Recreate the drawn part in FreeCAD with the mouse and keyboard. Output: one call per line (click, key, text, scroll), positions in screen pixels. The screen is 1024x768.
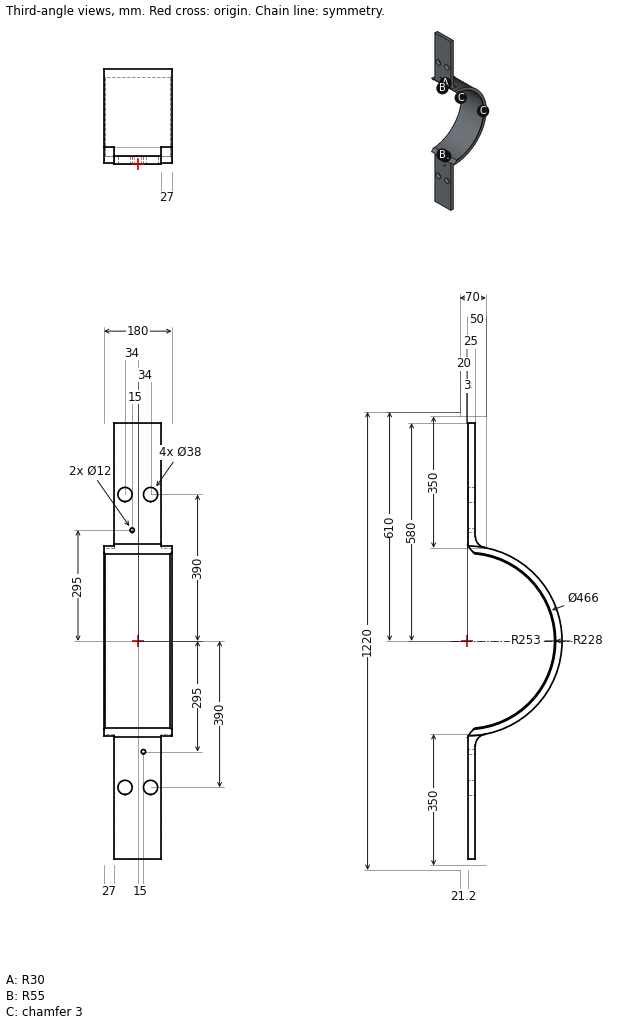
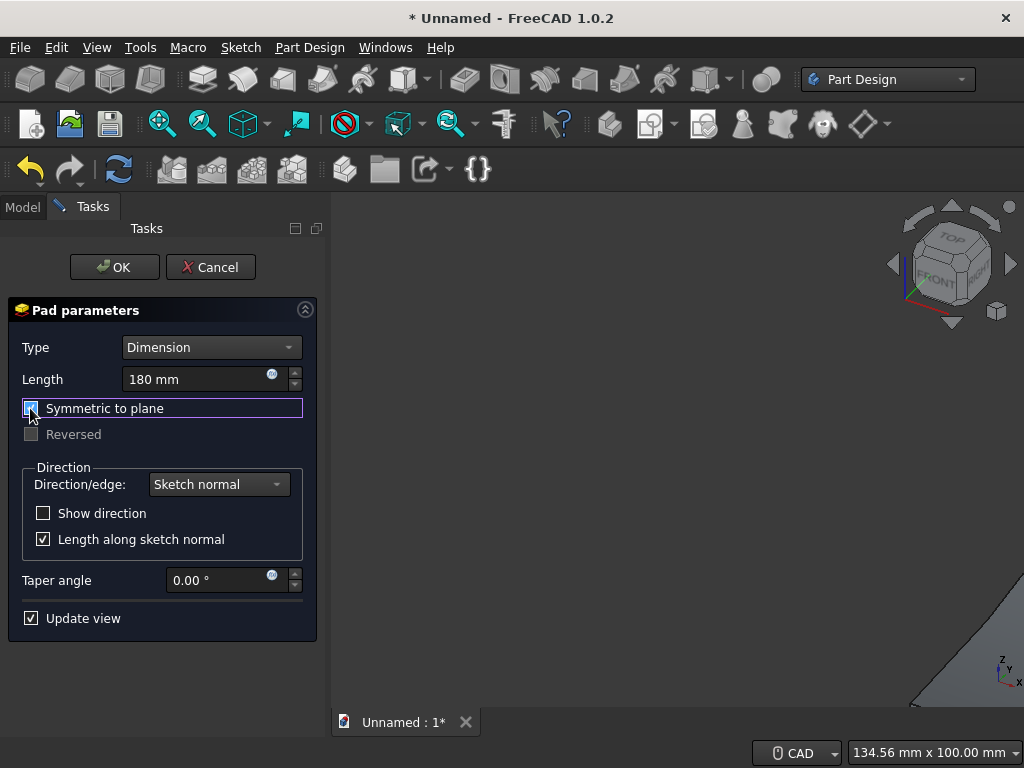
click(115, 267)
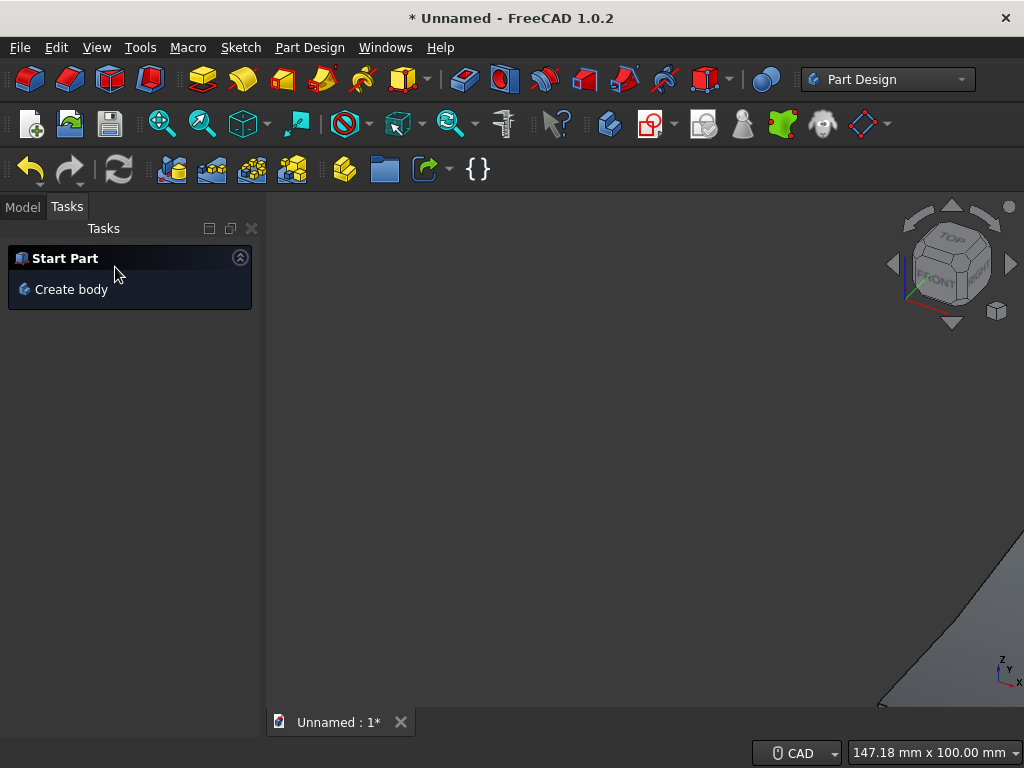
click(164, 124)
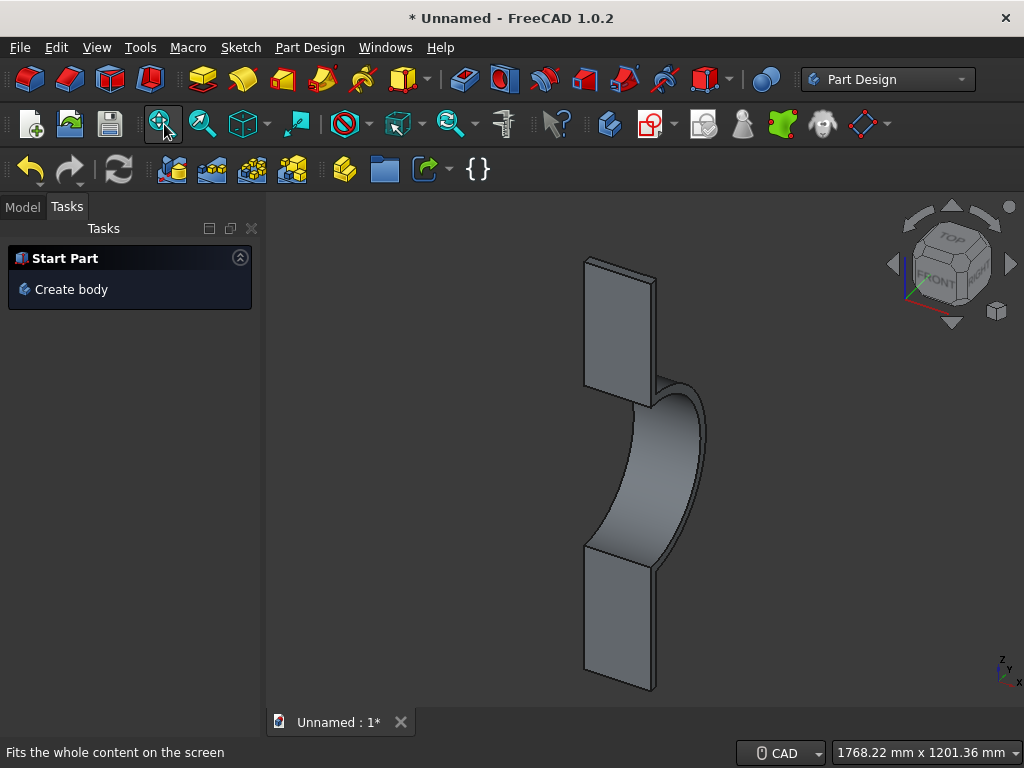
key(0)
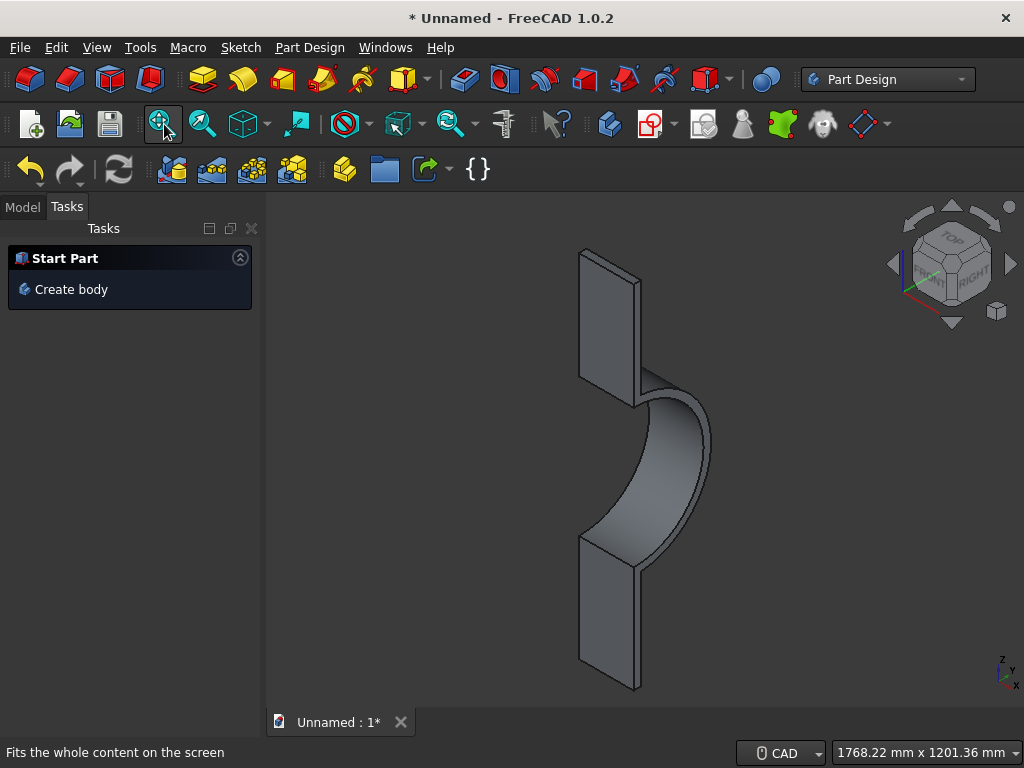
key(2)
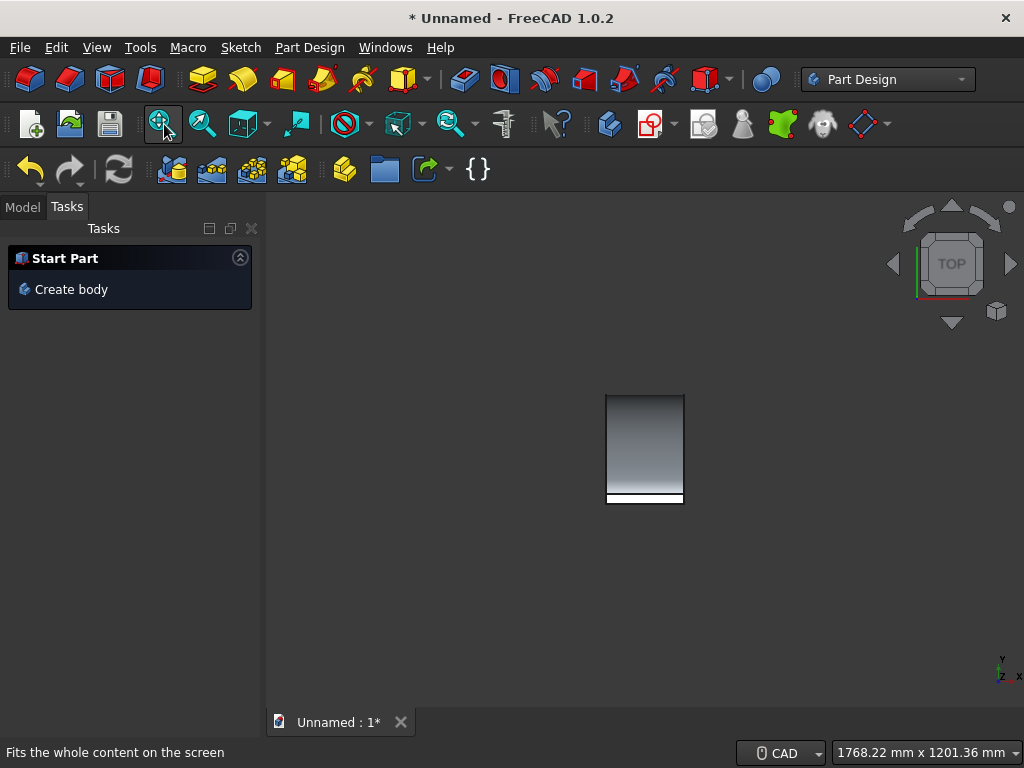
click(164, 124)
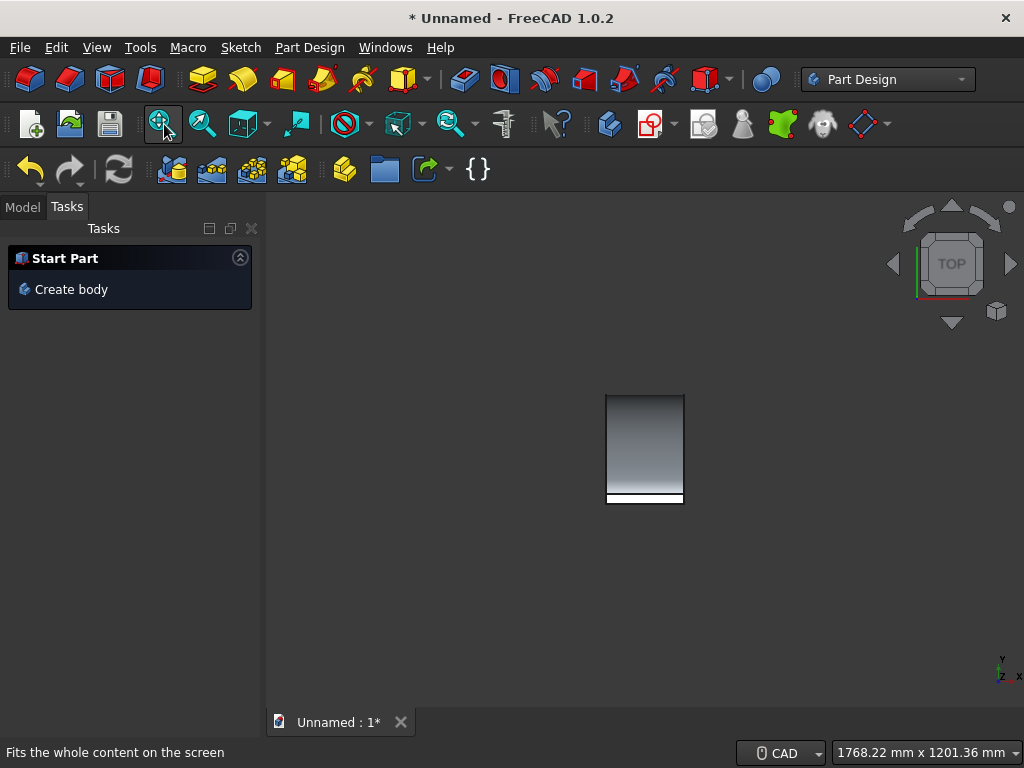
key(1)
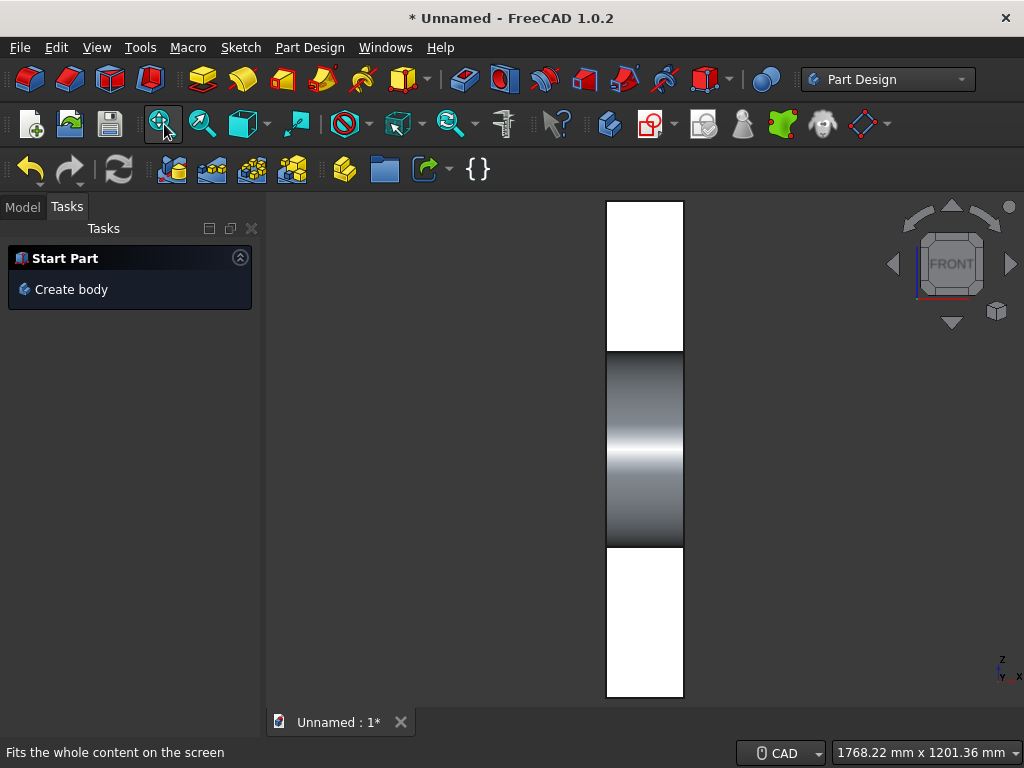
key(3)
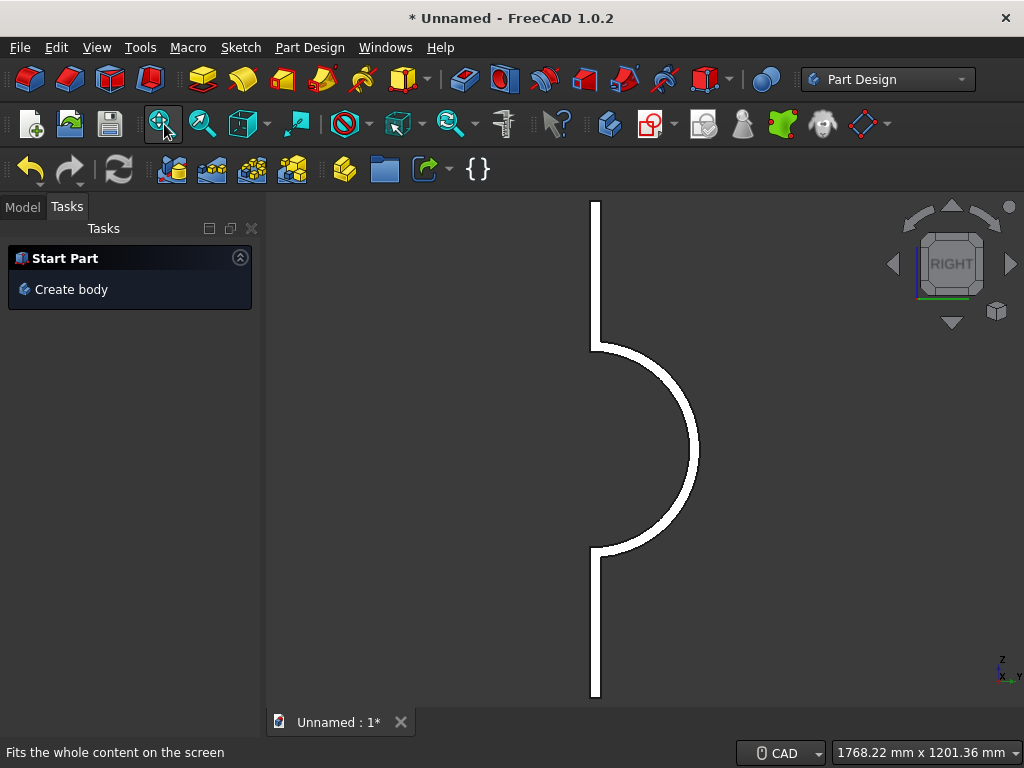
key(5)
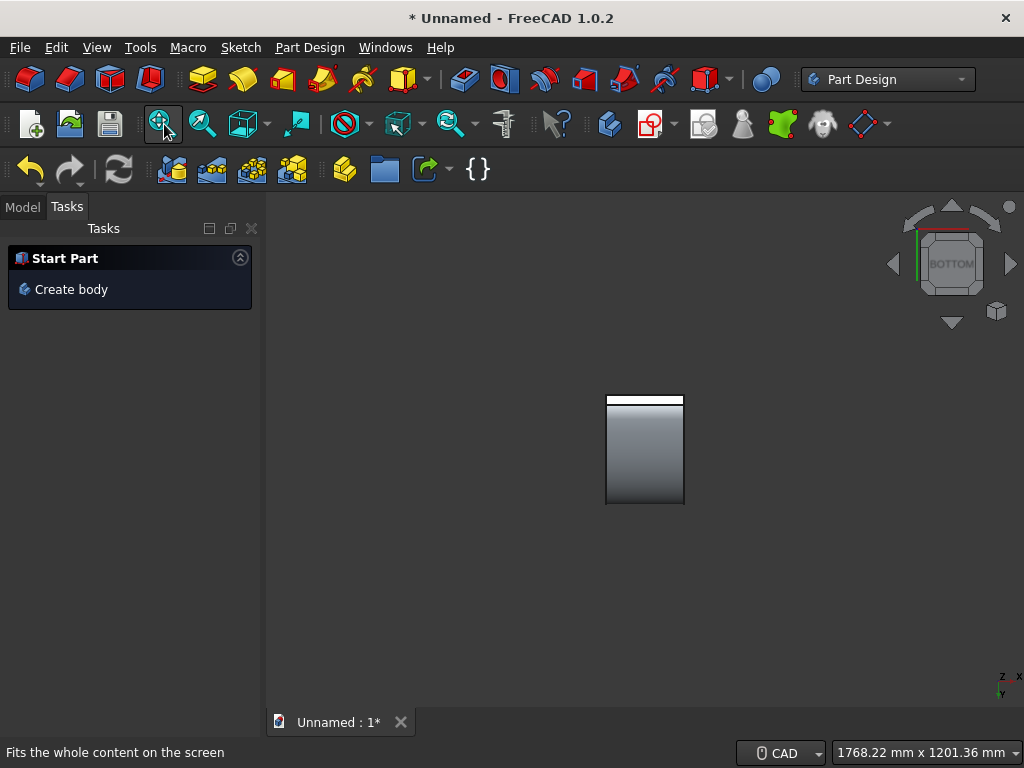
click(164, 124)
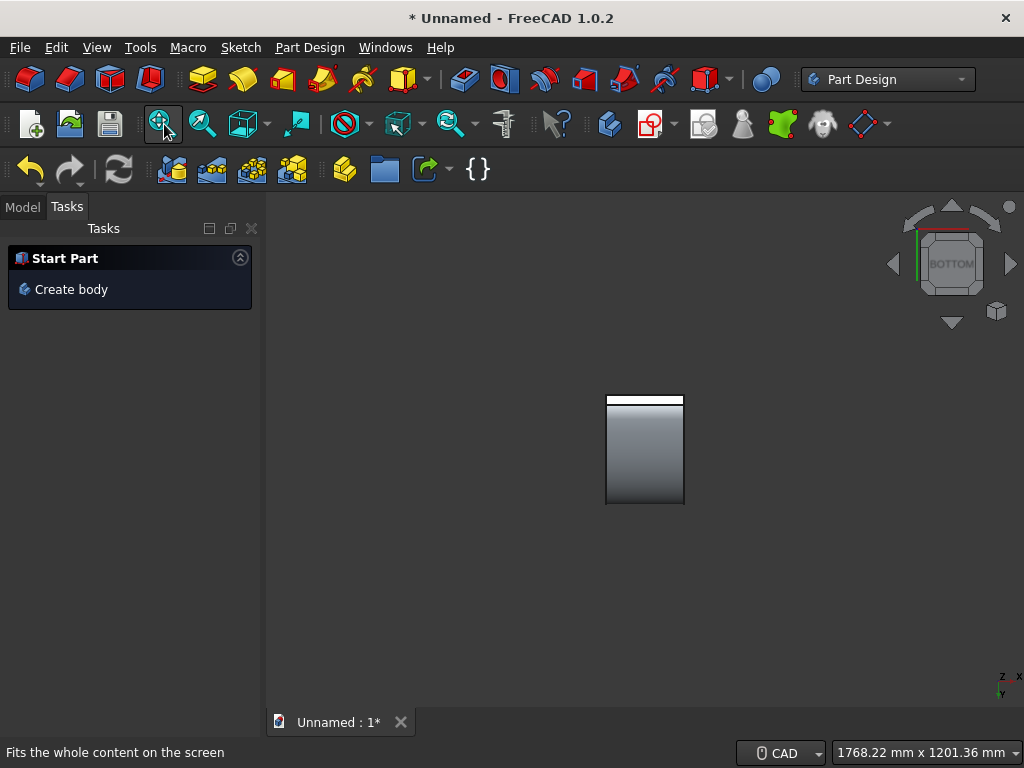
key(4)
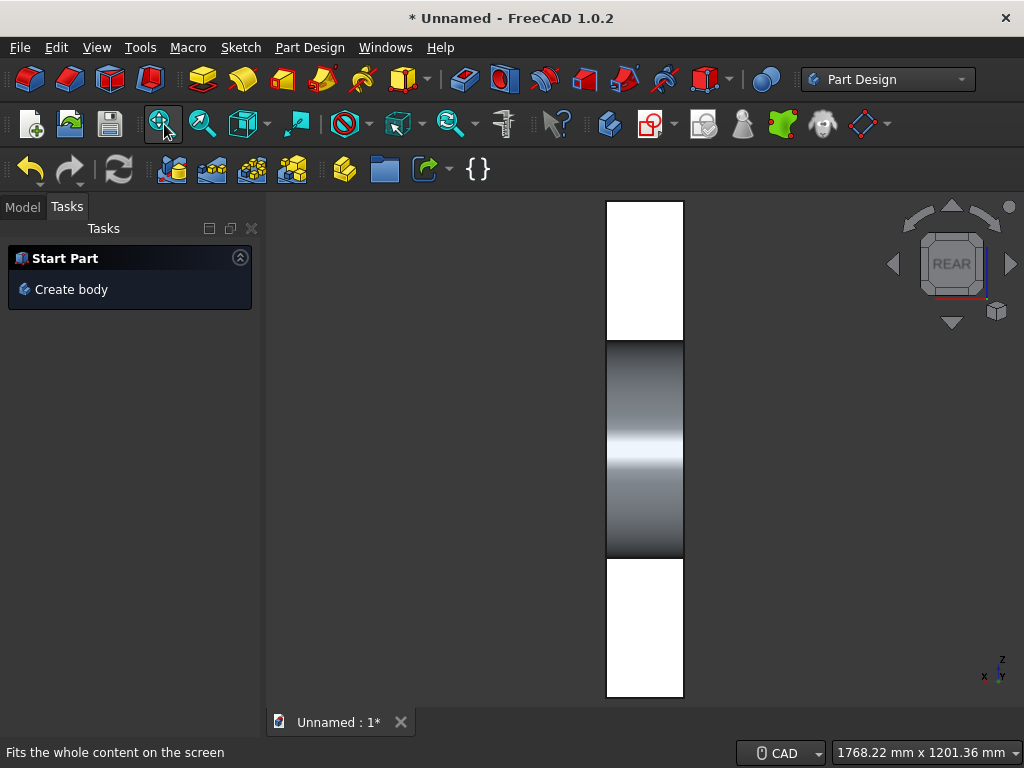
key(6)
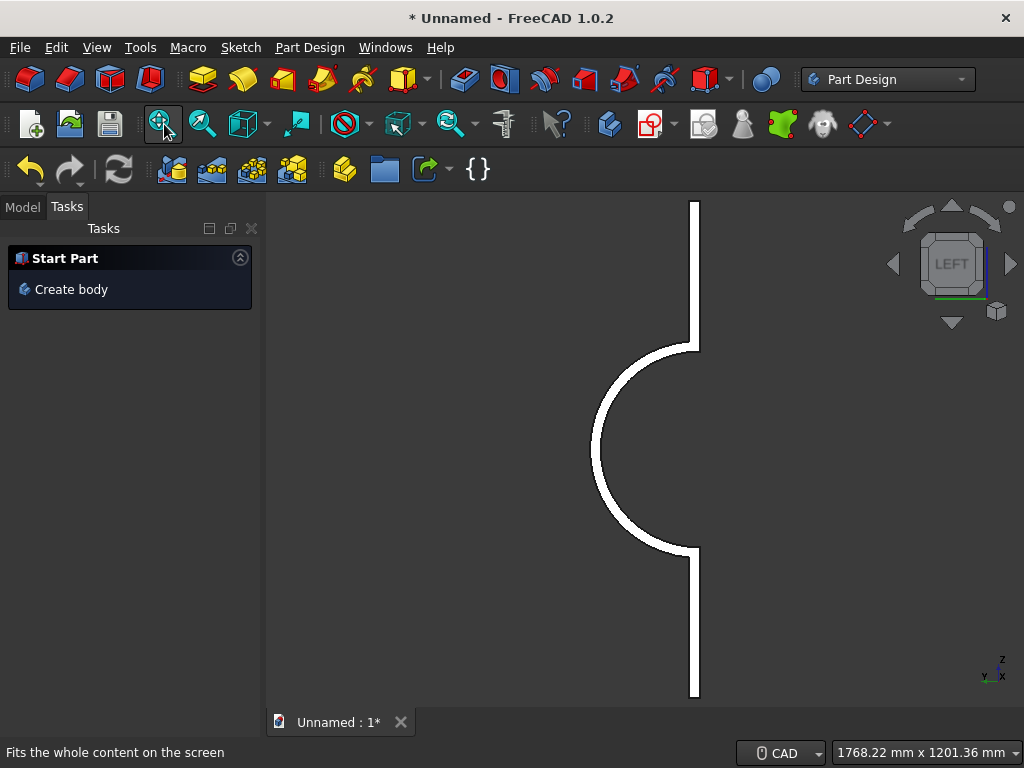
key(v)
key(3)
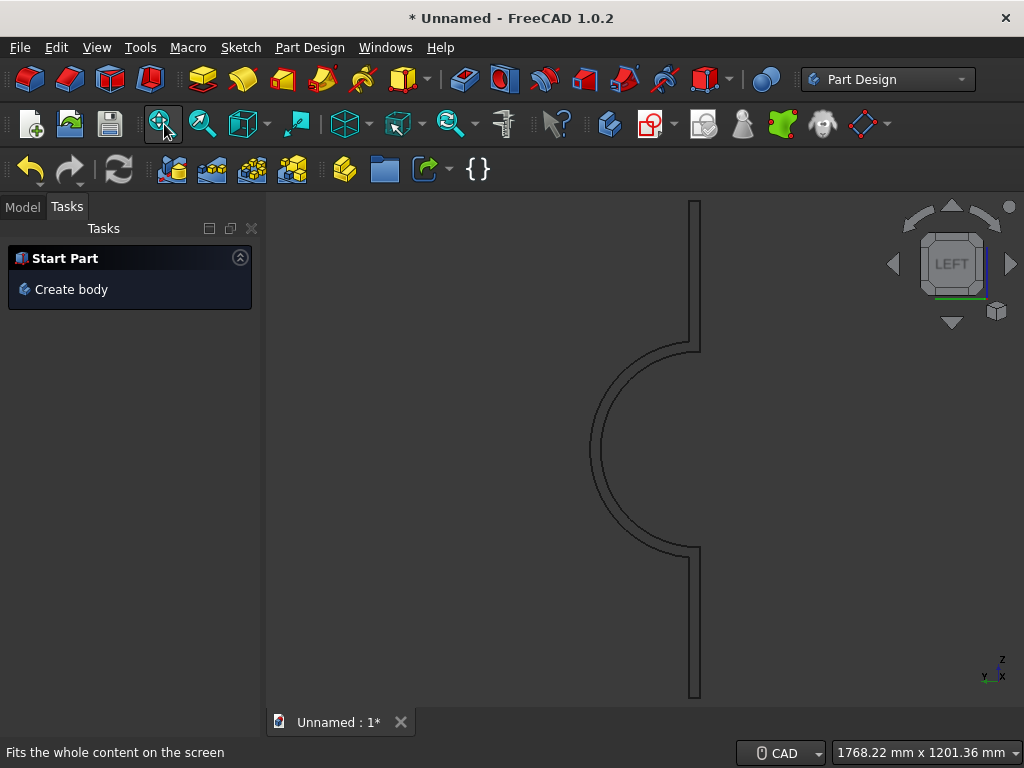
key(0)